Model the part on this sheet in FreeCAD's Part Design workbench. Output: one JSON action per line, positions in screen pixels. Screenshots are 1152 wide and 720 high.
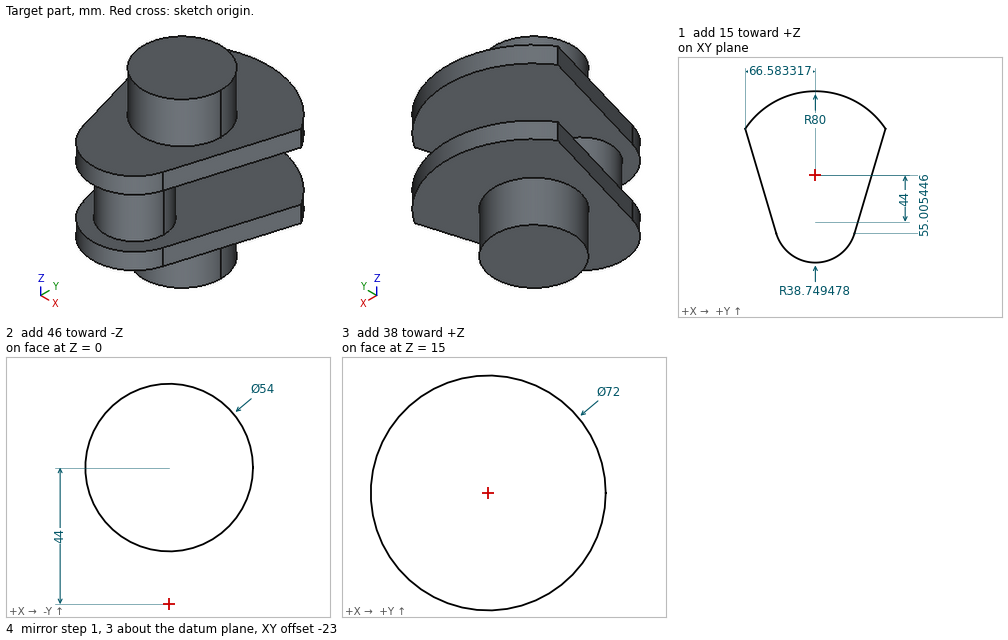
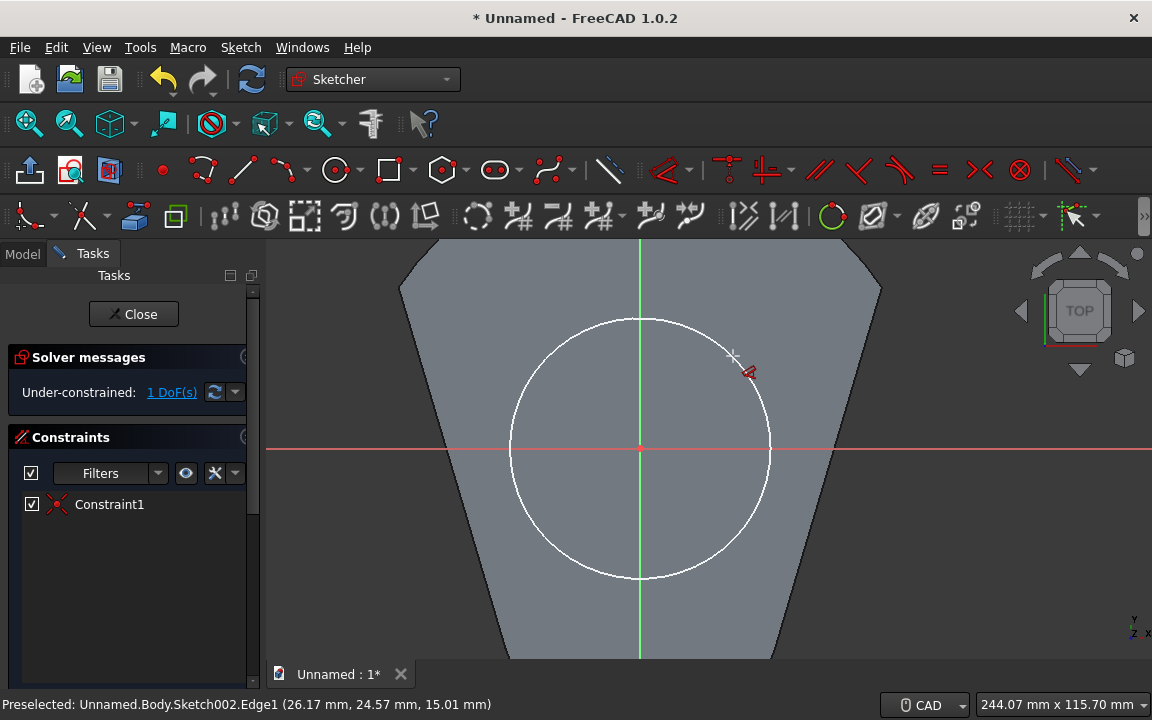
{"action": "left_click", "coordinate": [732, 356]}
{"action": "left_click", "coordinate": [755, 333]}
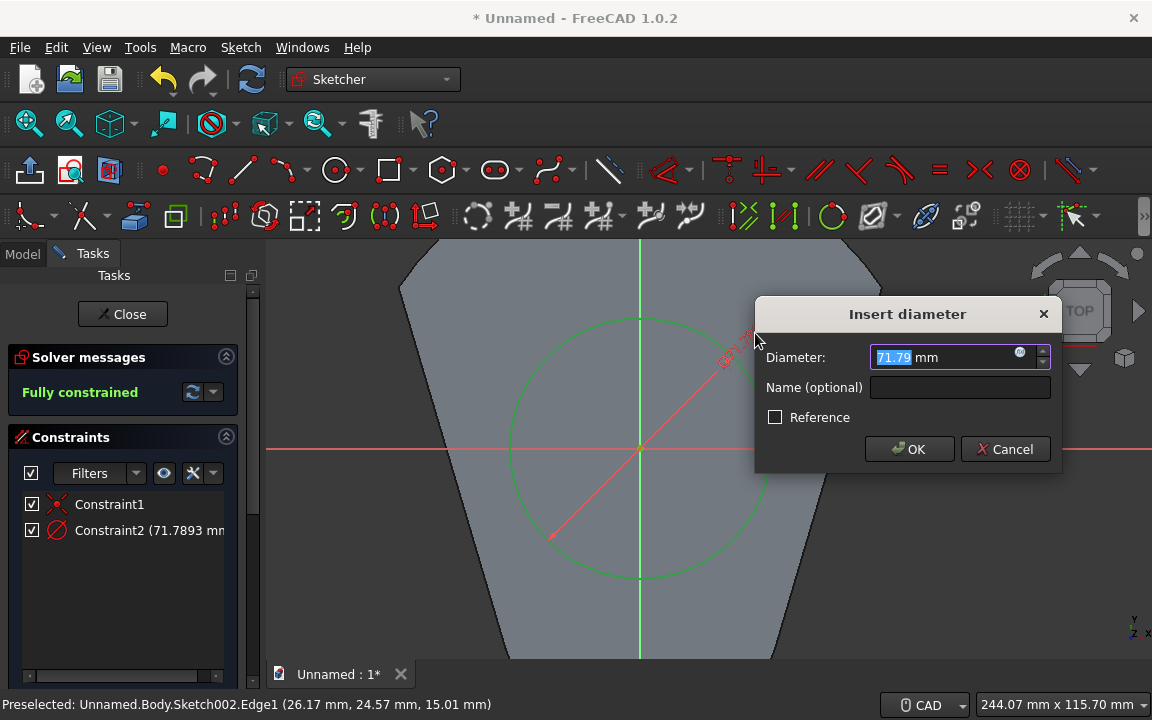
{"action": "type", "text": "72"}
{"action": "key", "text": "Return"}
{"action": "key", "text": "Escape"}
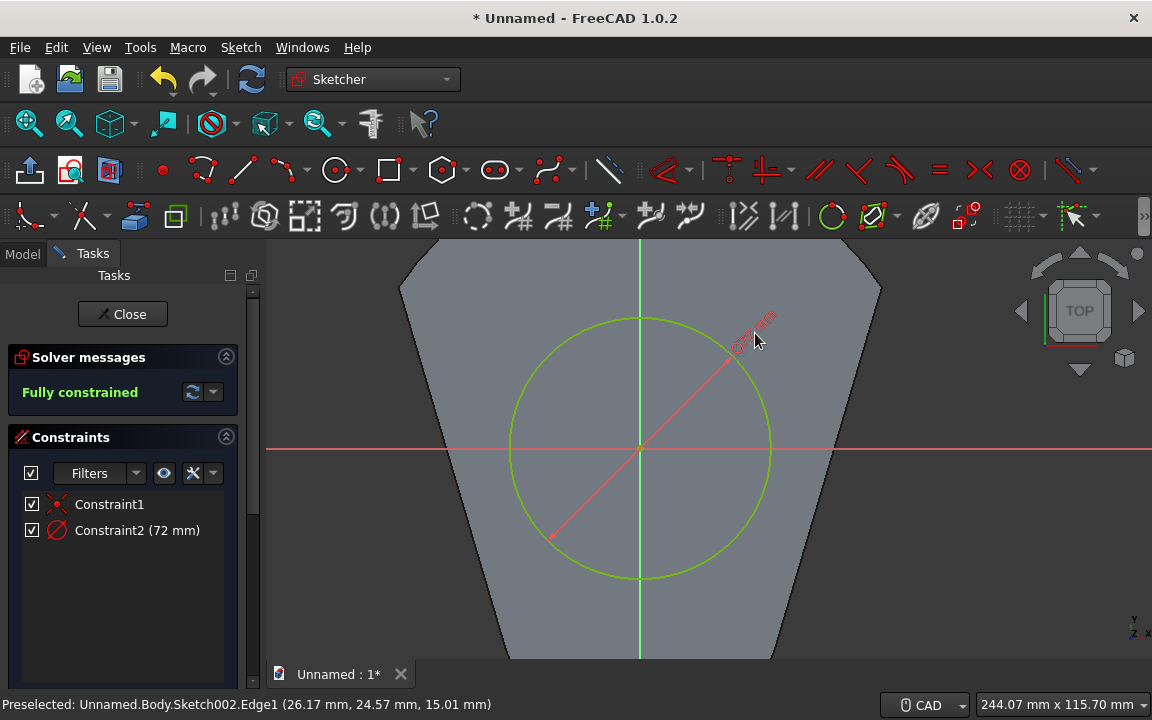
{"action": "left_click", "coordinate": [123, 314]}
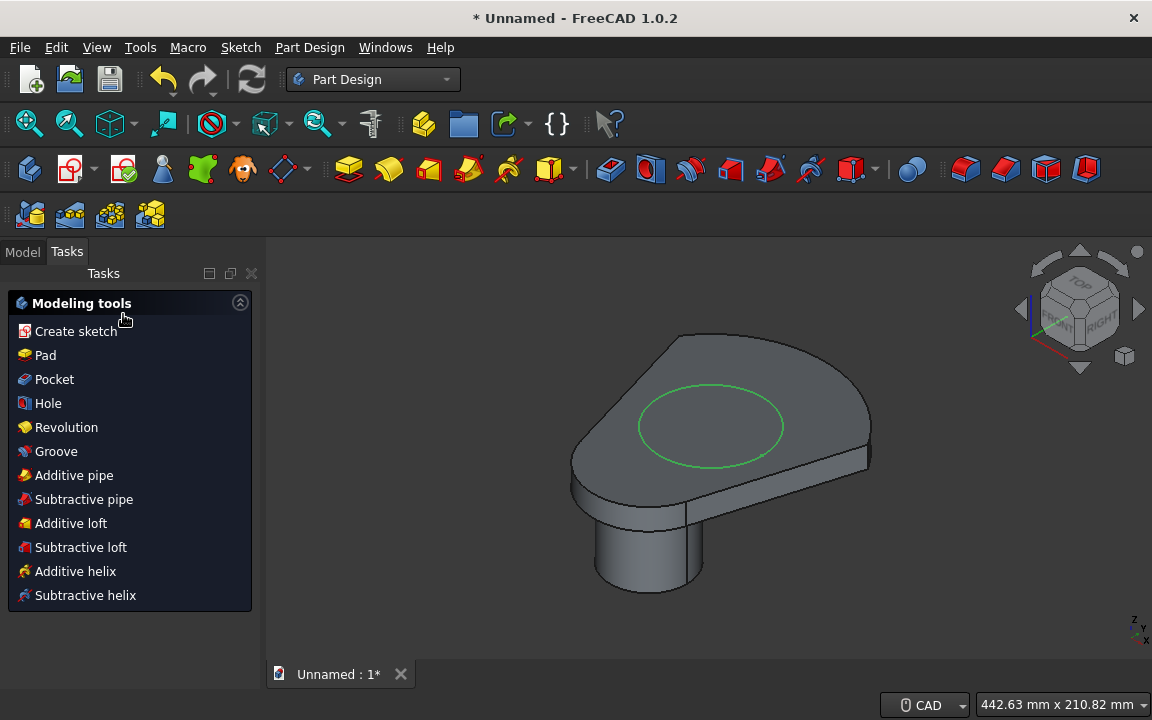
{"action": "left_click", "coordinate": [350, 170]}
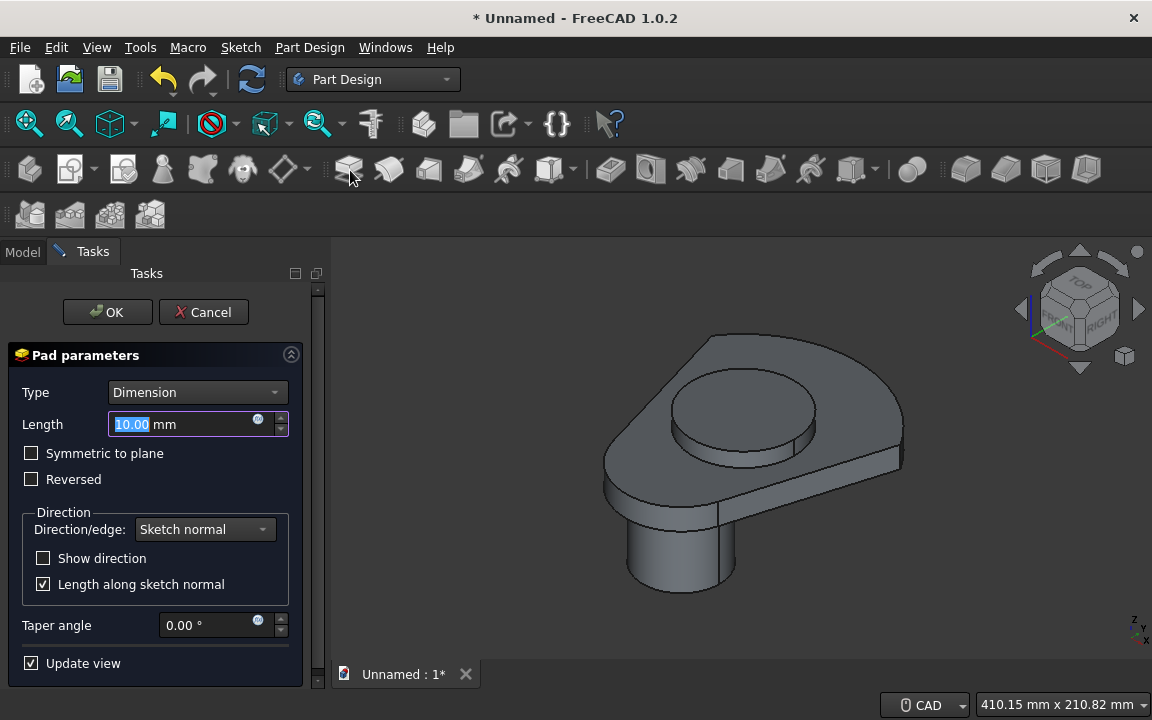
{"action": "type", "text": "38"}
{"action": "key", "text": "Tab"}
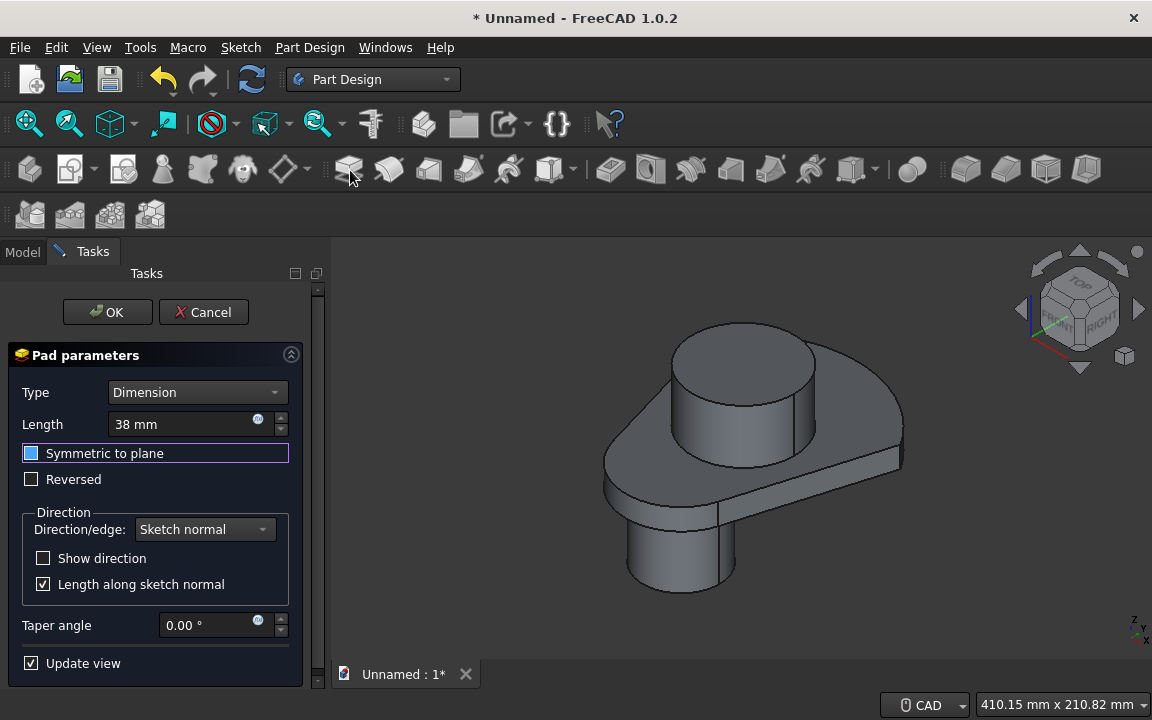
{"action": "left_click", "coordinate": [108, 312]}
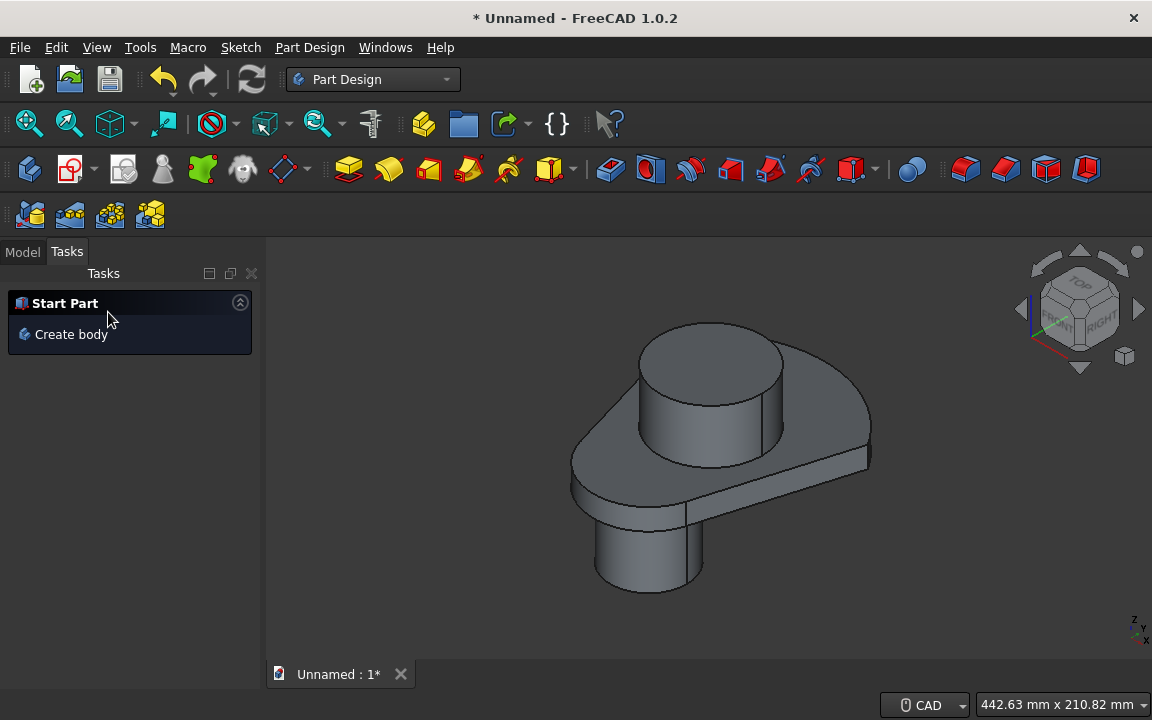
{"action": "left_click", "coordinate": [23, 251]}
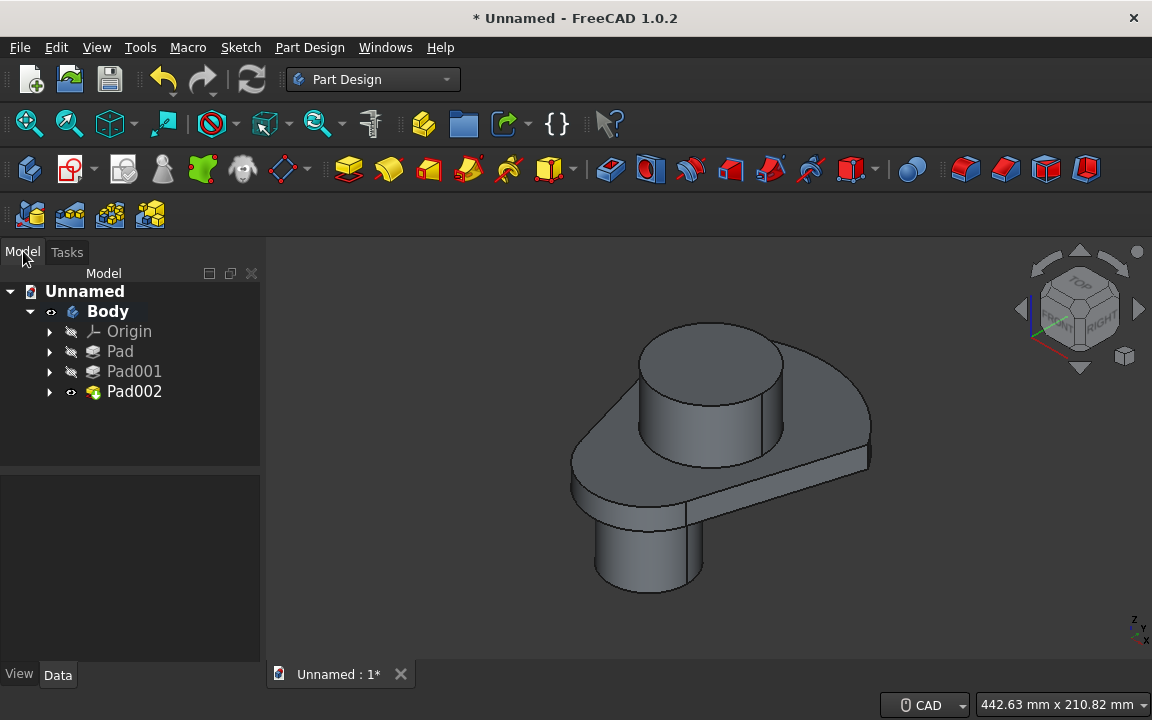
{"action": "left_click", "coordinate": [50, 332]}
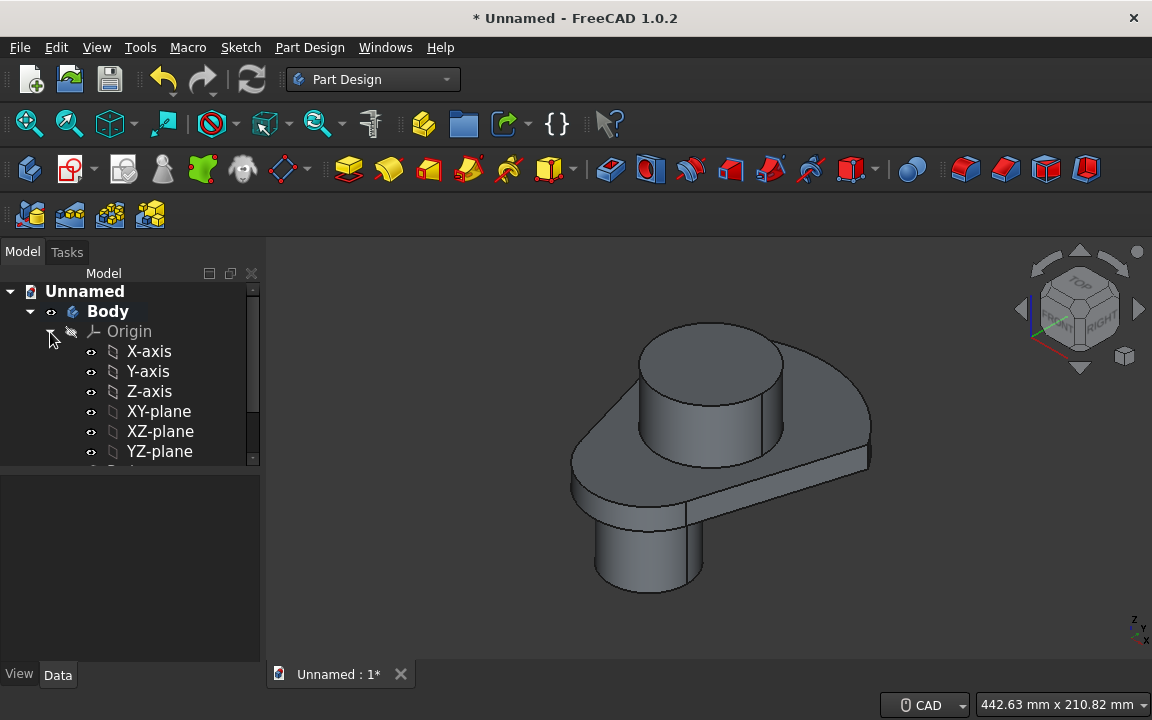
{"action": "left_click", "coordinate": [136, 412]}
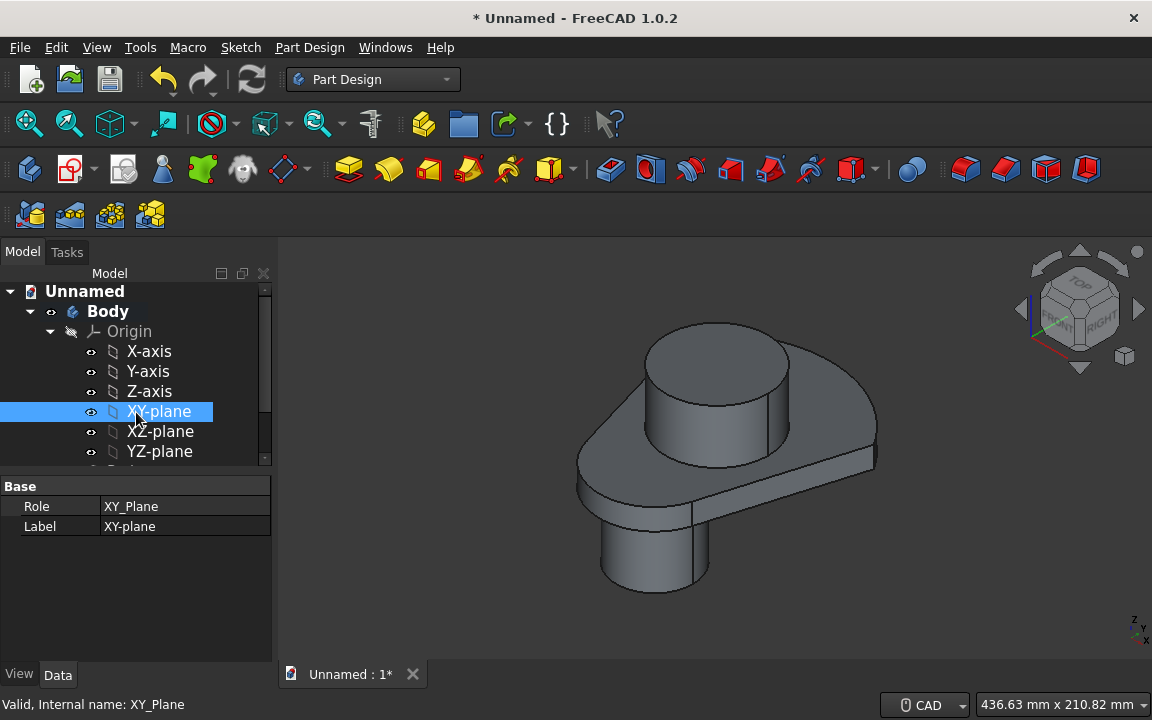
{"action": "left_click", "coordinate": [284, 170]}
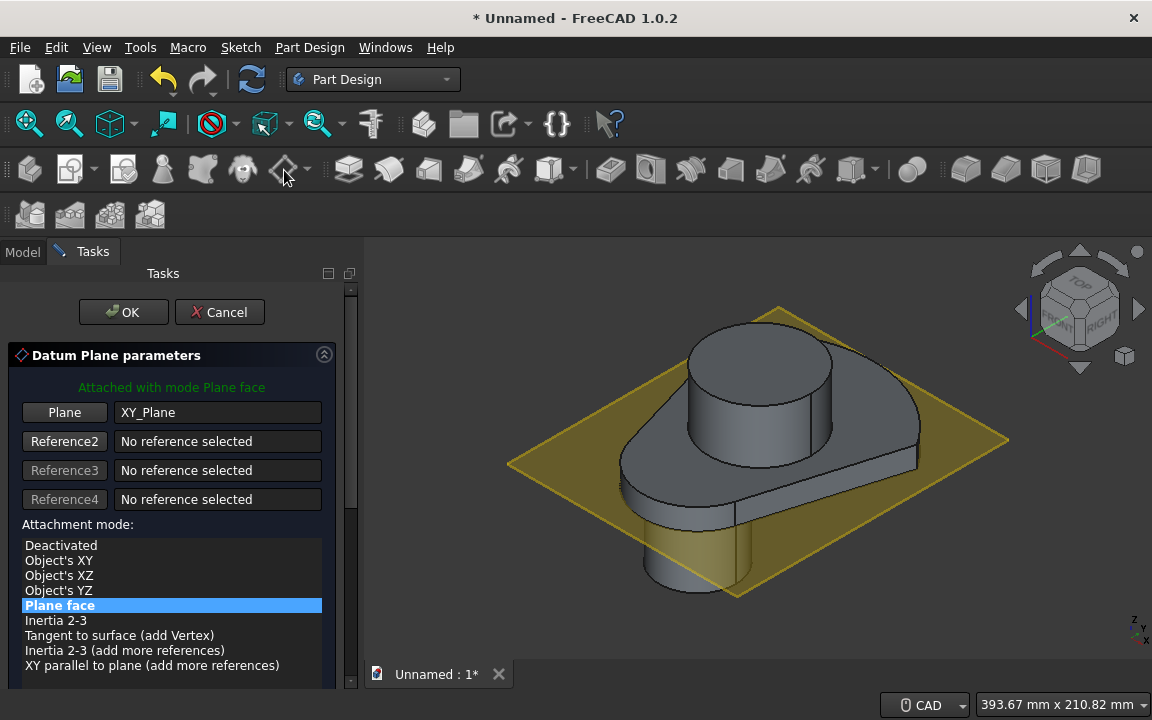
{"action": "scroll", "coordinate": [351, 486], "scroll_direction": "down", "scroll_amount": 4}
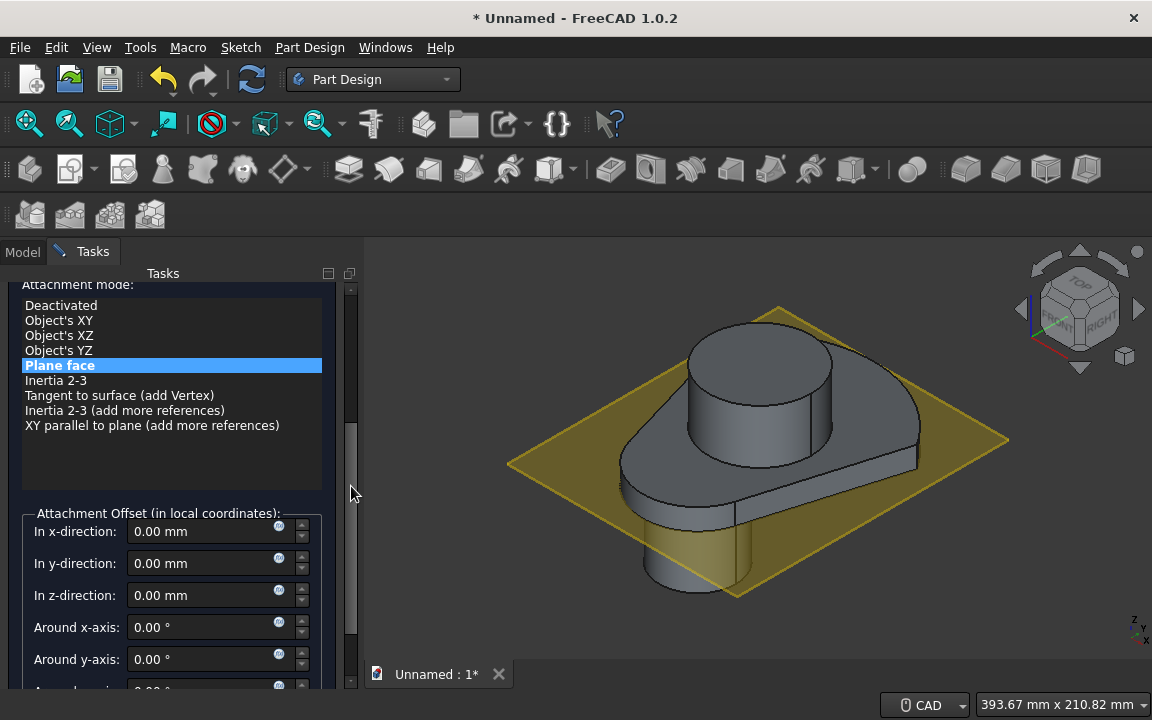
{"action": "triple_click", "coordinate": [210, 595]}